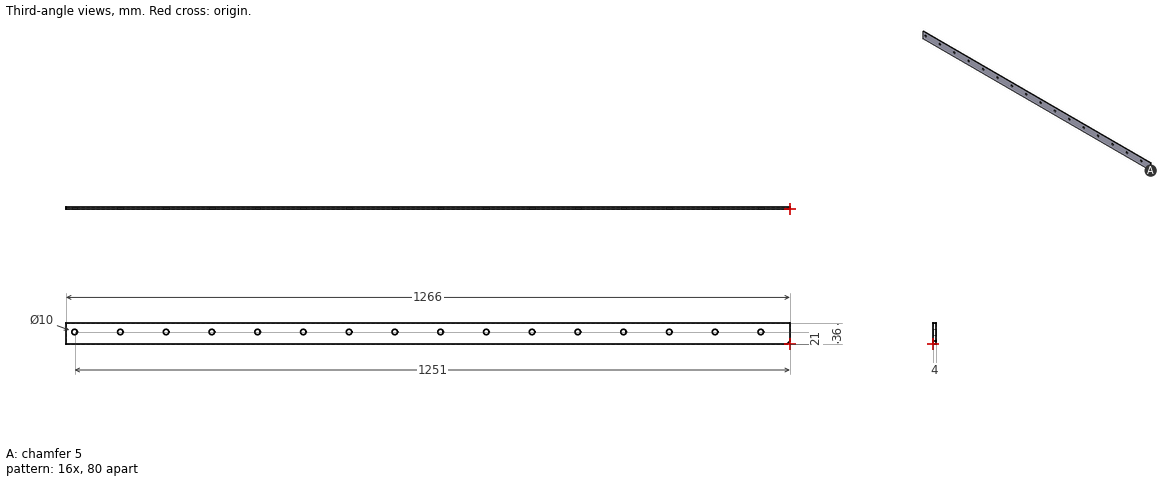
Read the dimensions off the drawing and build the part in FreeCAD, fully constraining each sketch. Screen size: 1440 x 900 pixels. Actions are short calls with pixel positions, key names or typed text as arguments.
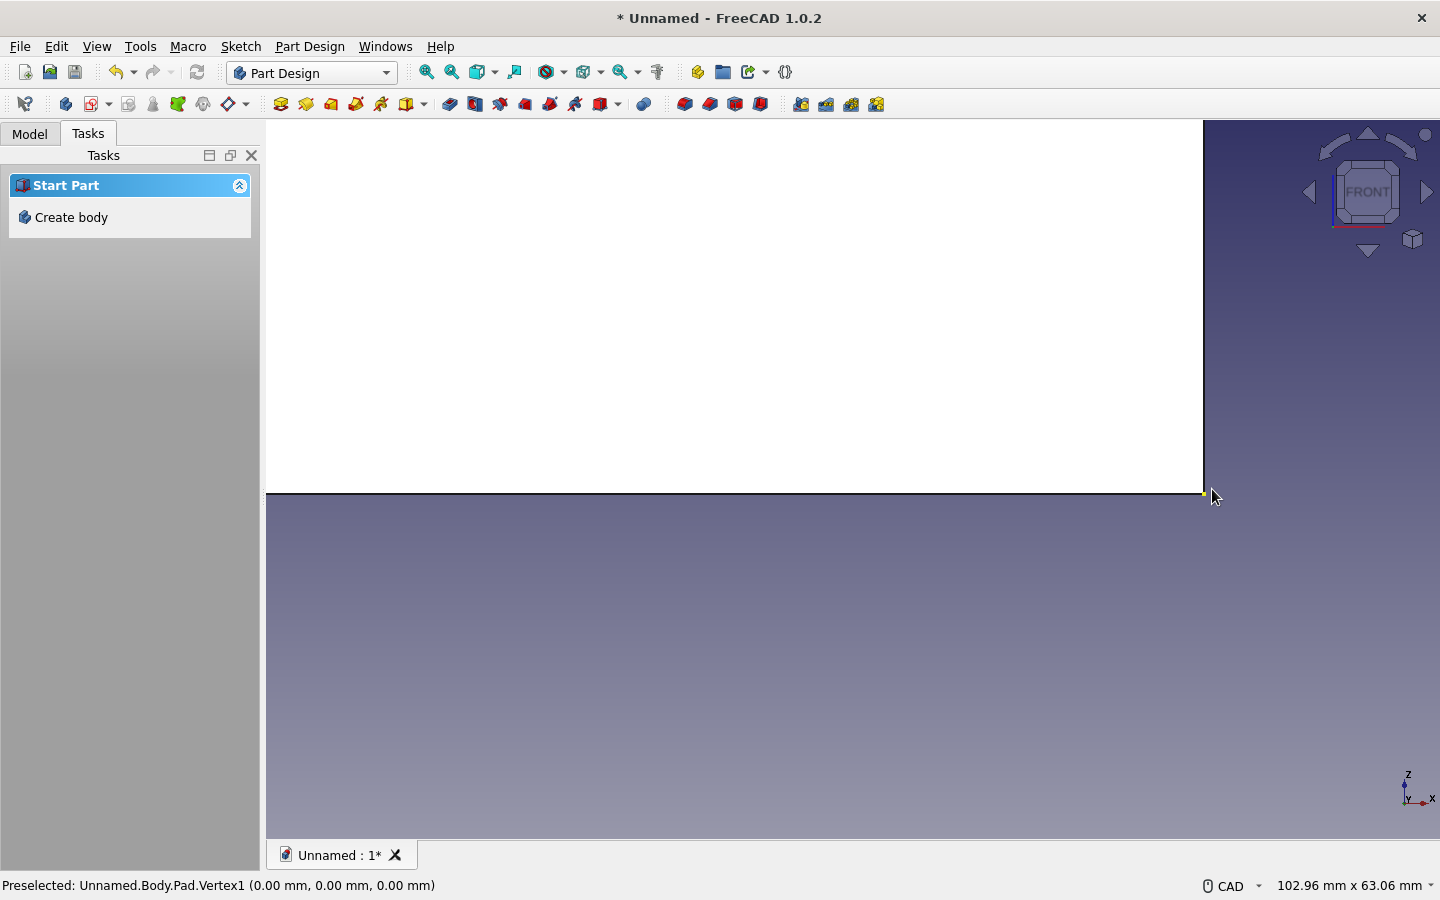
click(427, 72)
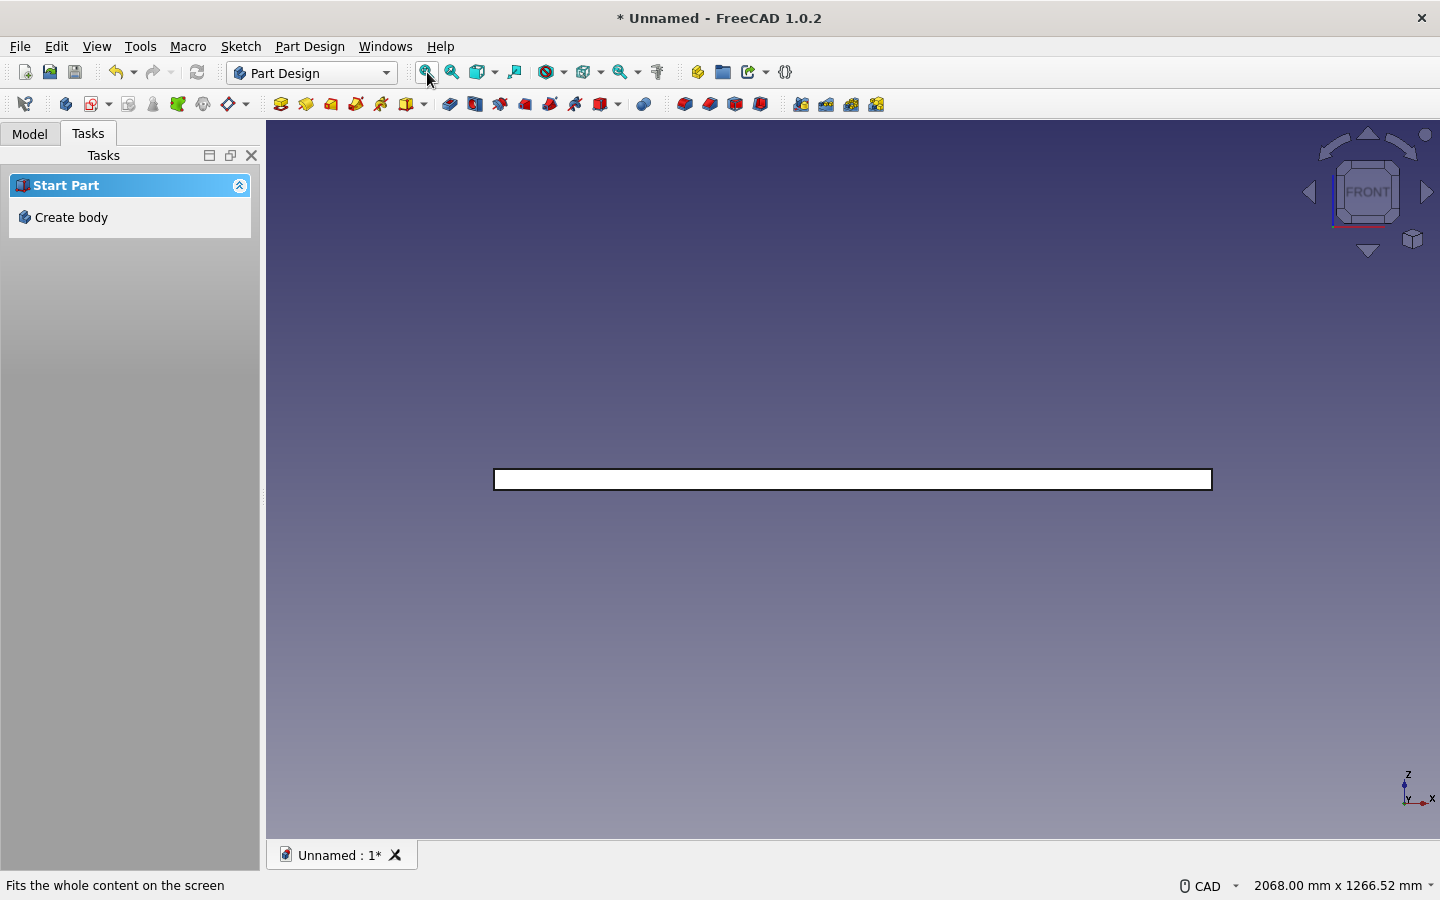
key(3)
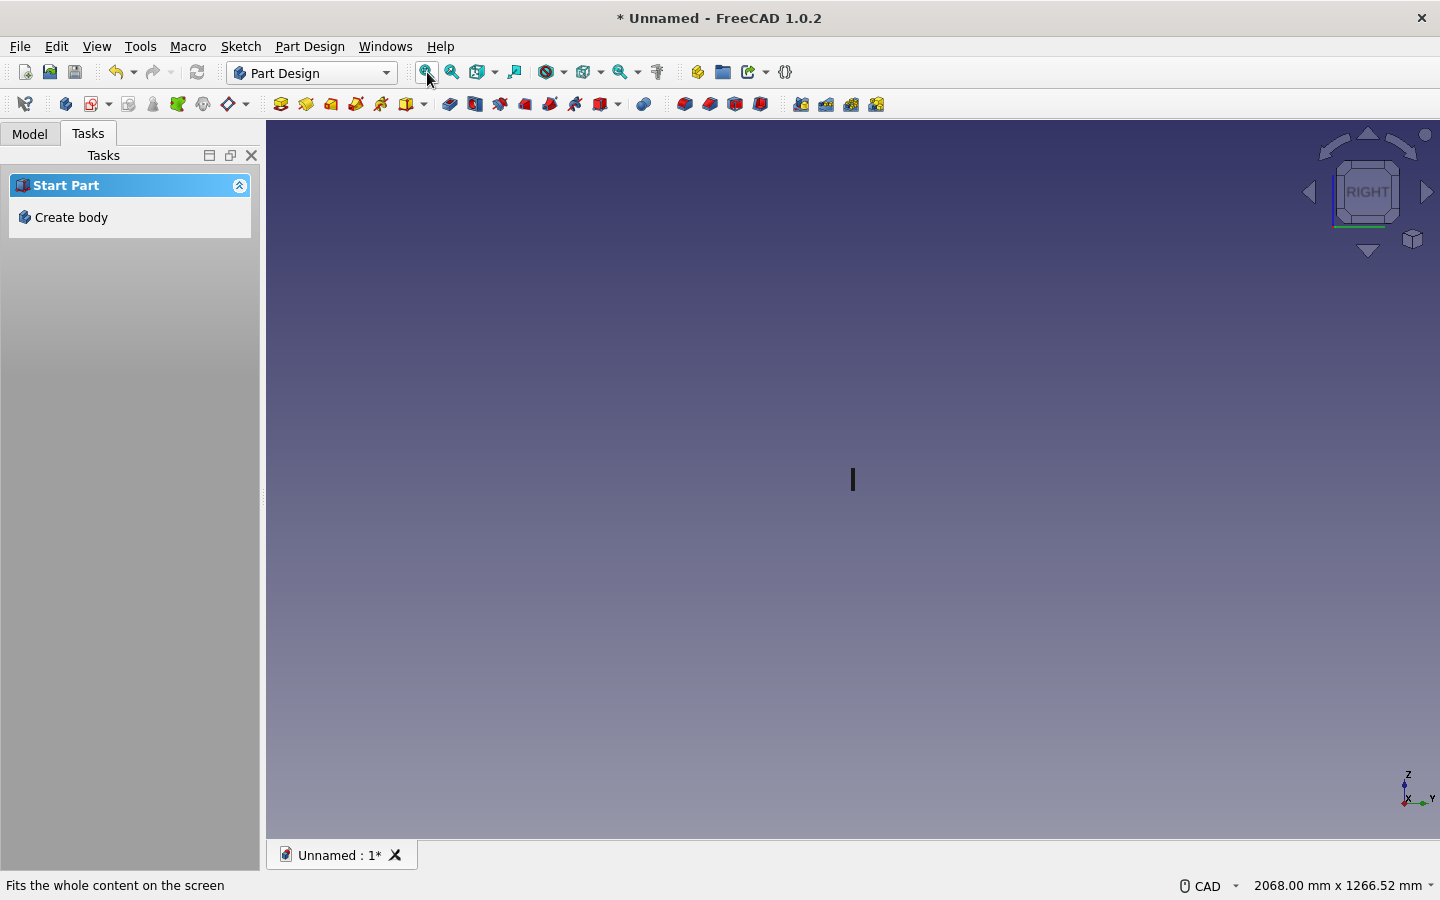
click(427, 72)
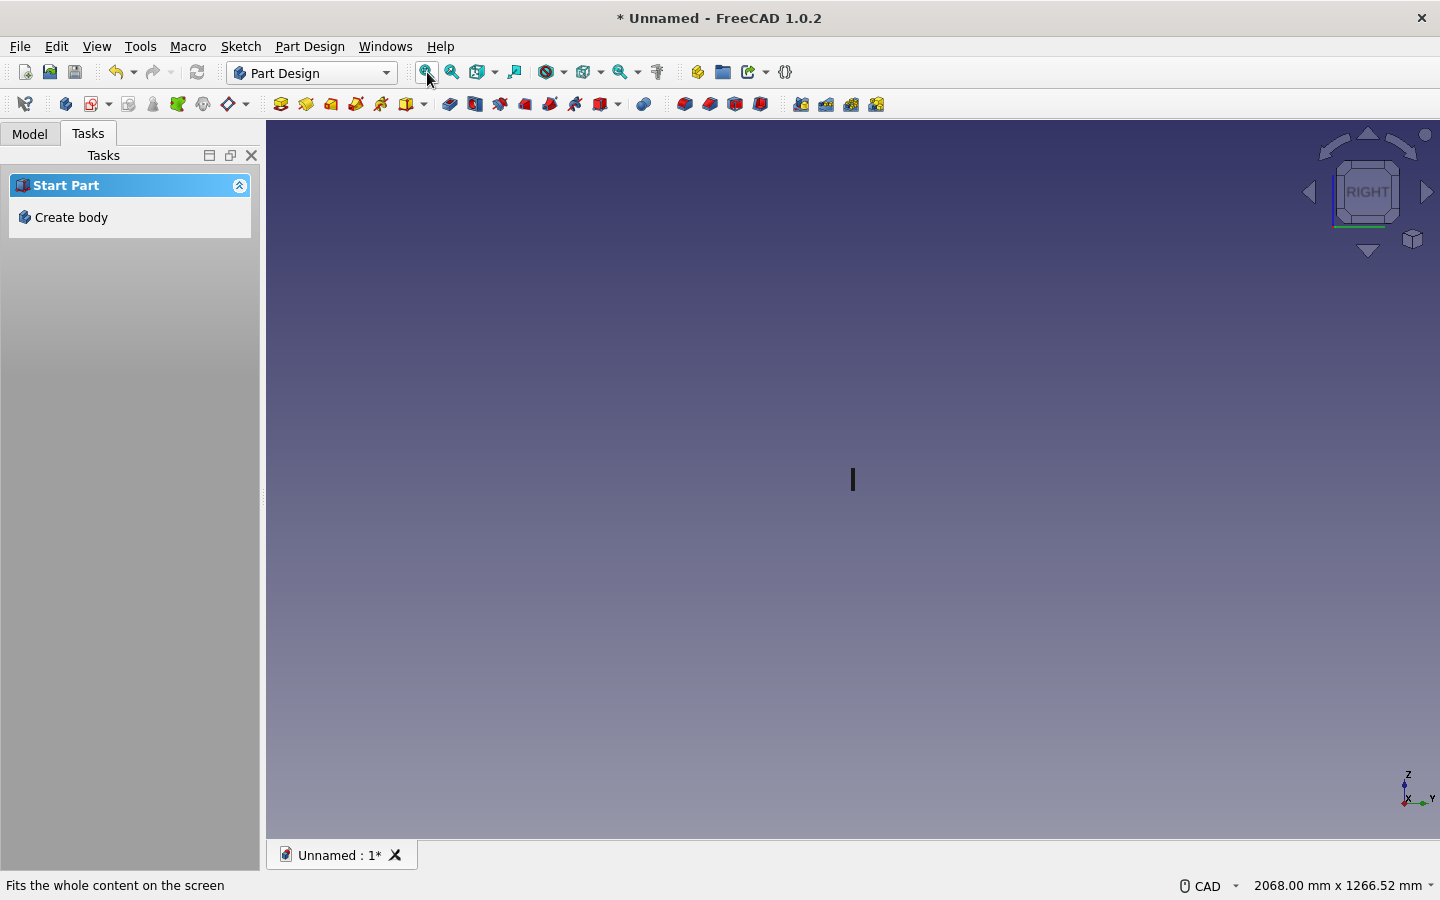
scroll(853, 489, up, 15)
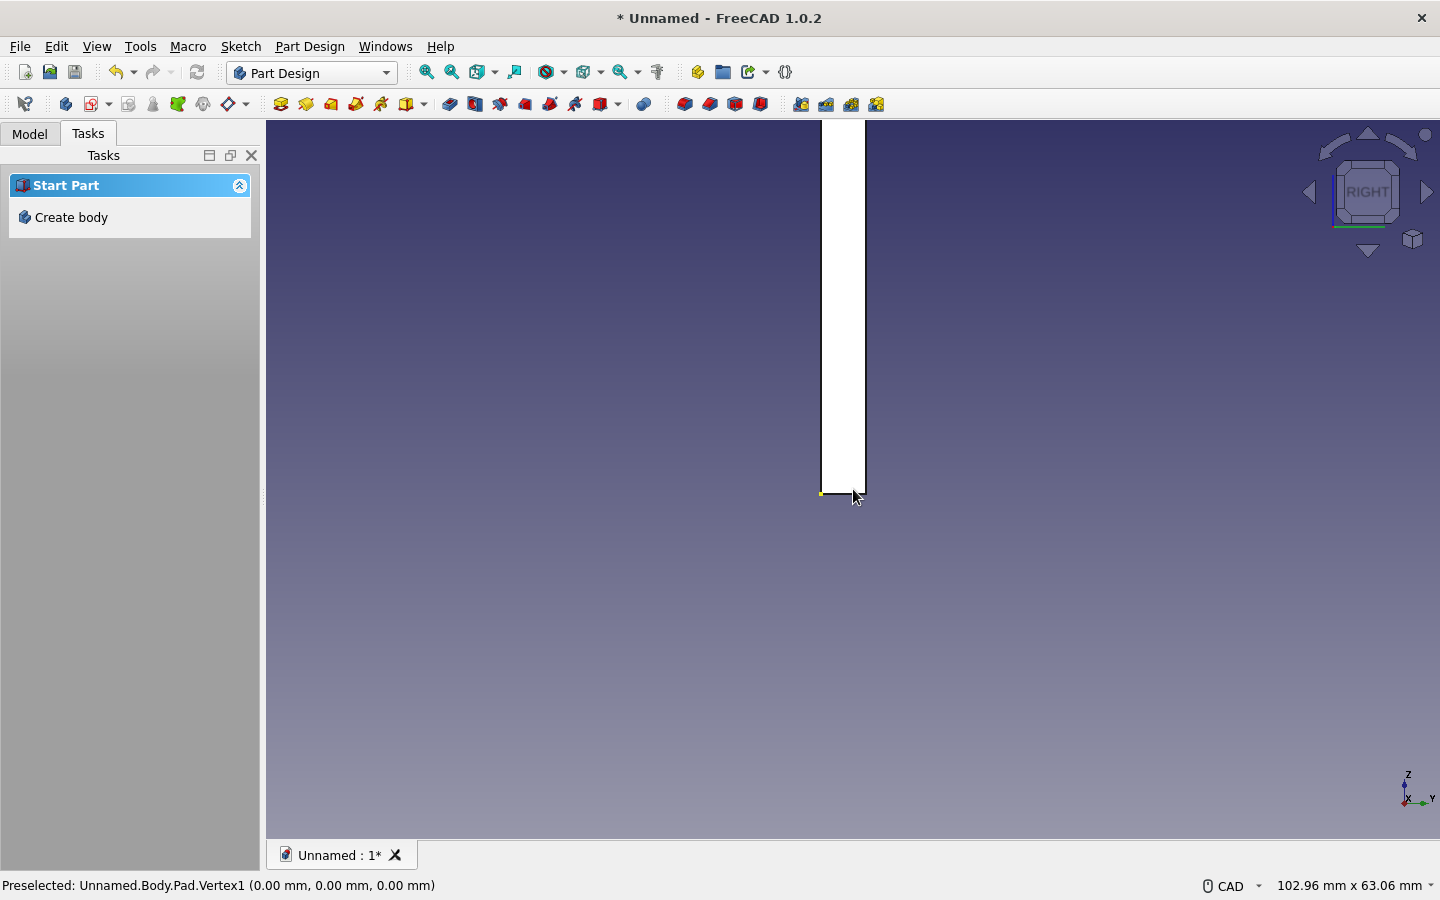
click(843, 493)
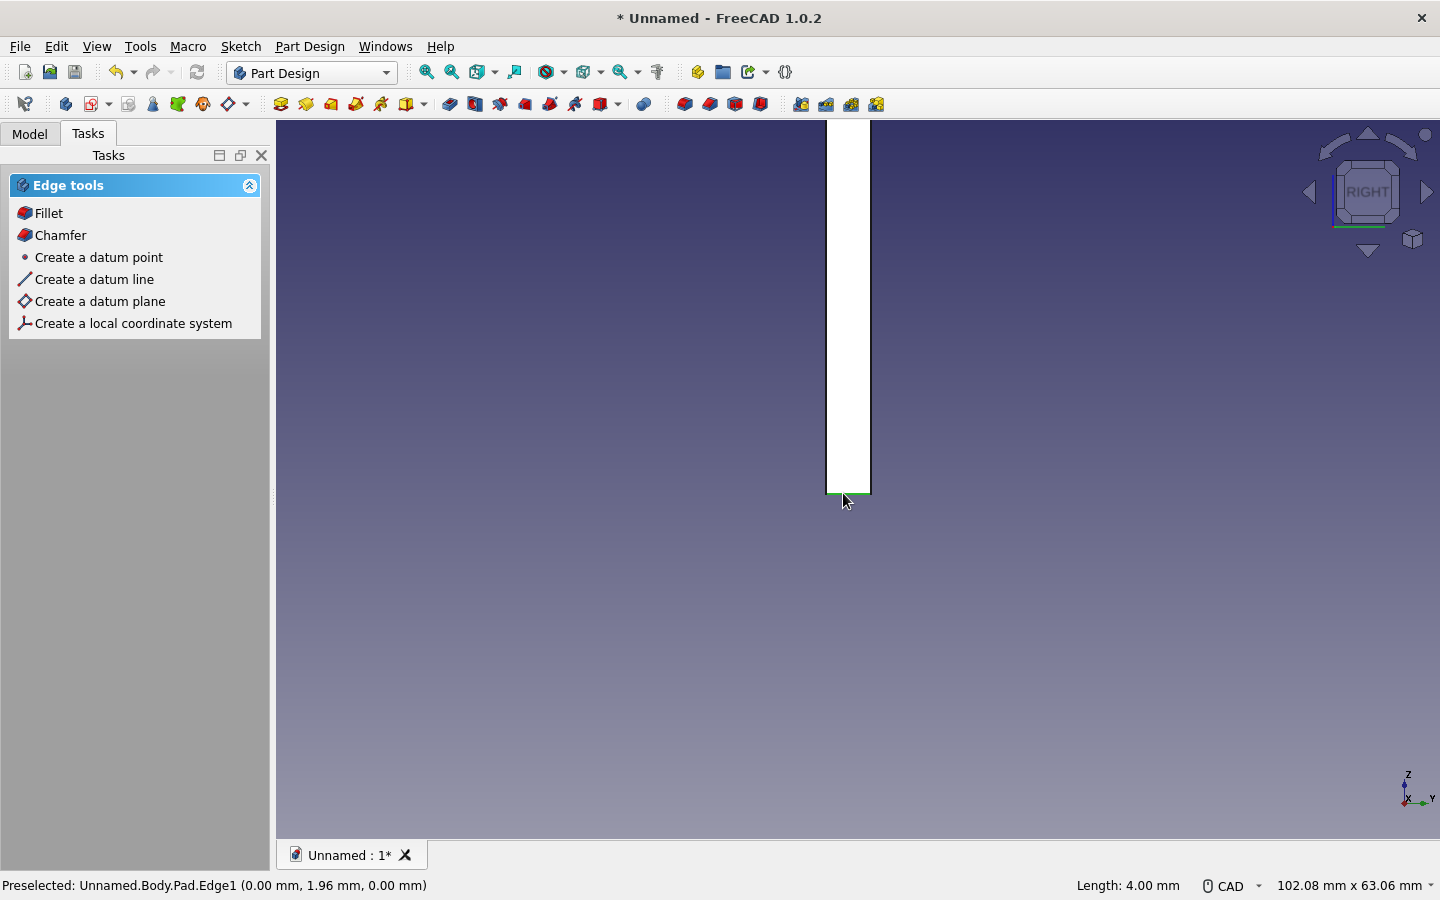
click(710, 104)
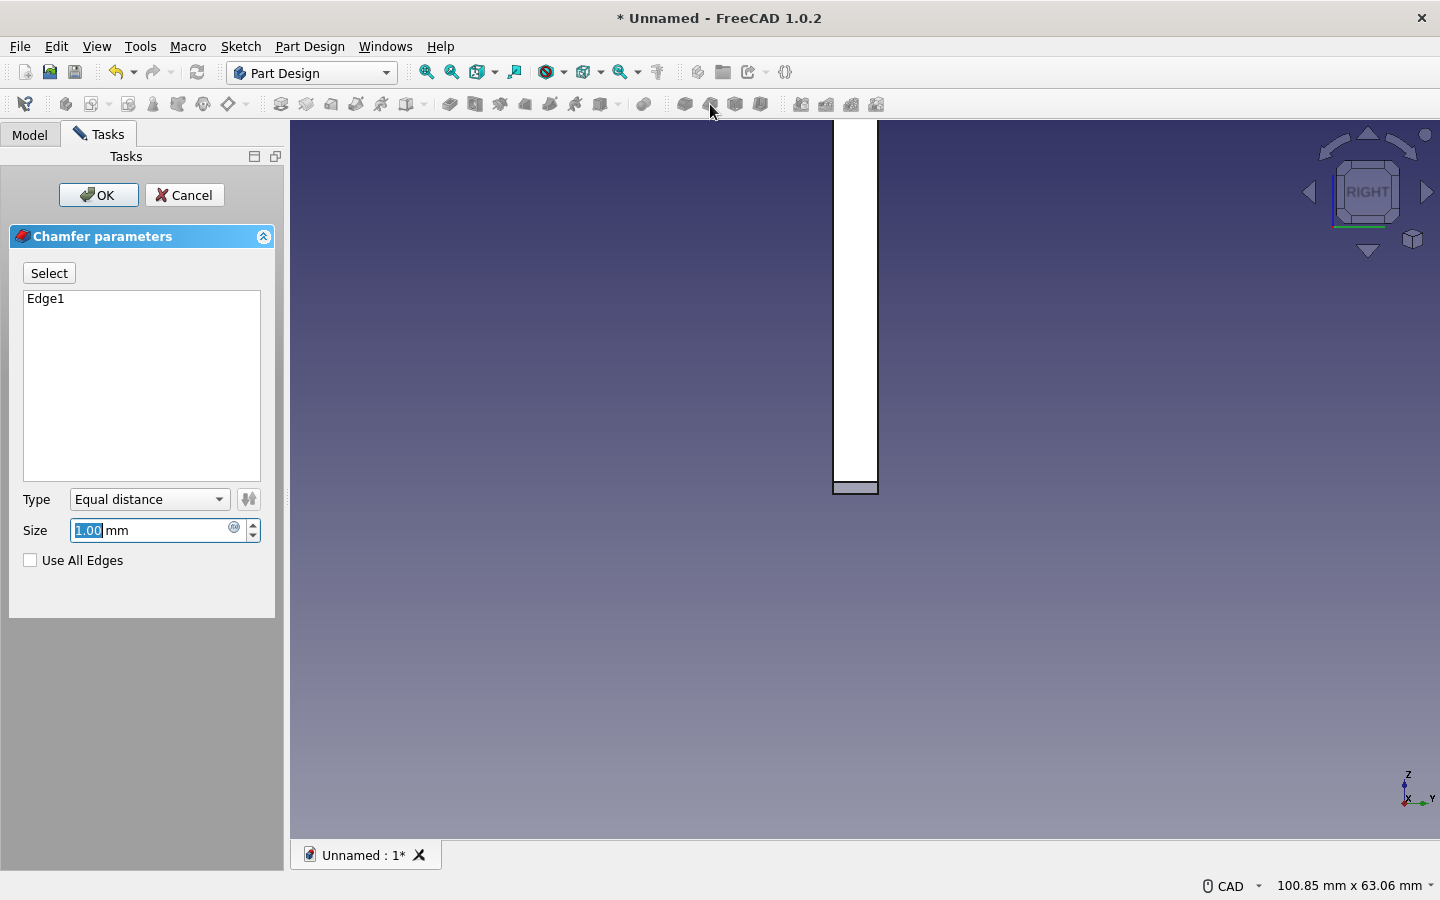
text(5)
key(Tab)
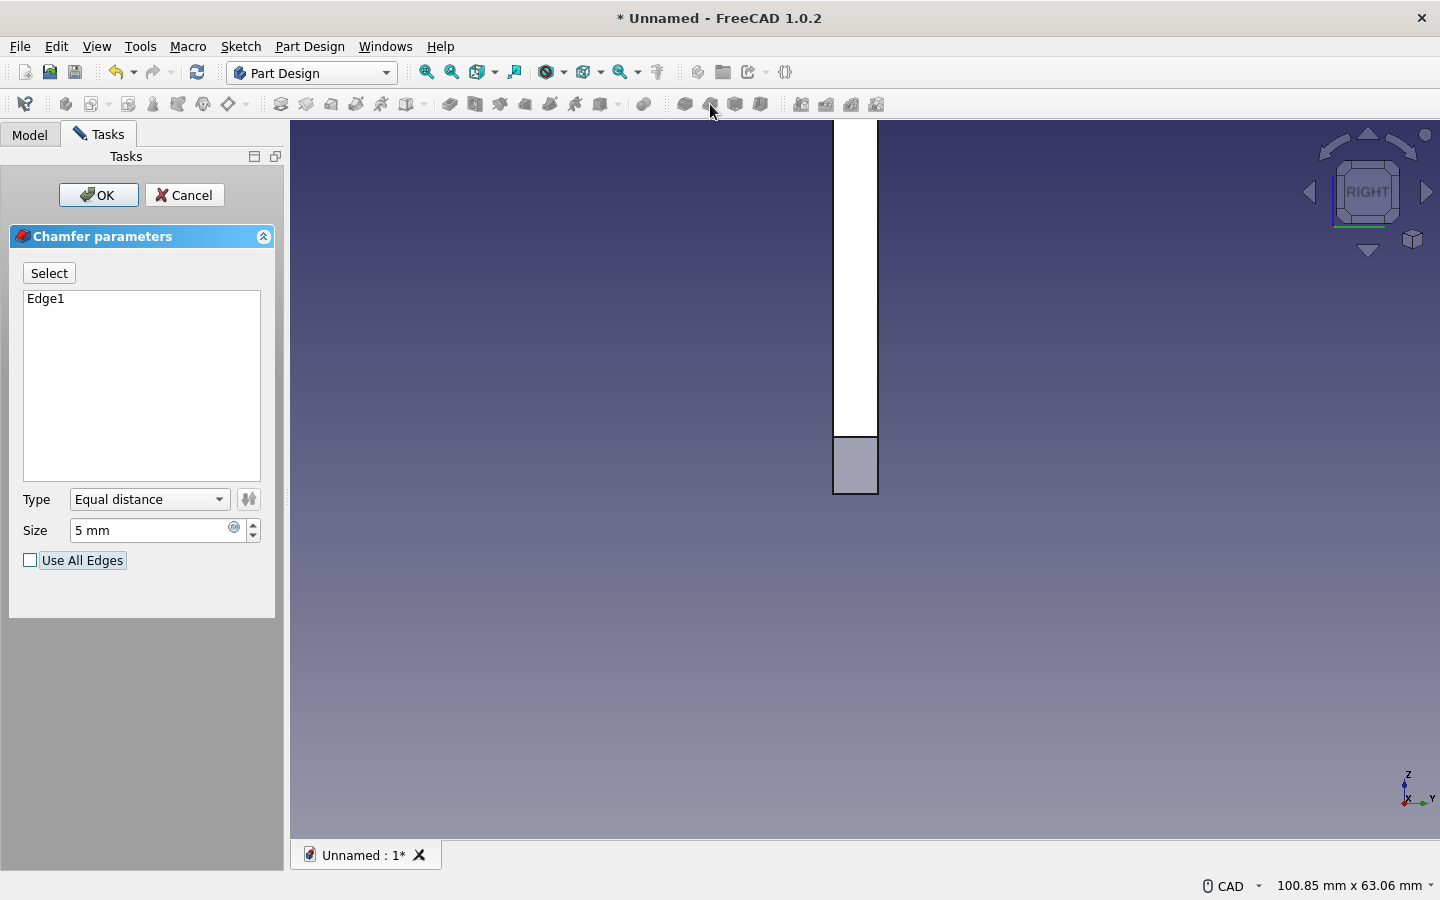
click(99, 195)